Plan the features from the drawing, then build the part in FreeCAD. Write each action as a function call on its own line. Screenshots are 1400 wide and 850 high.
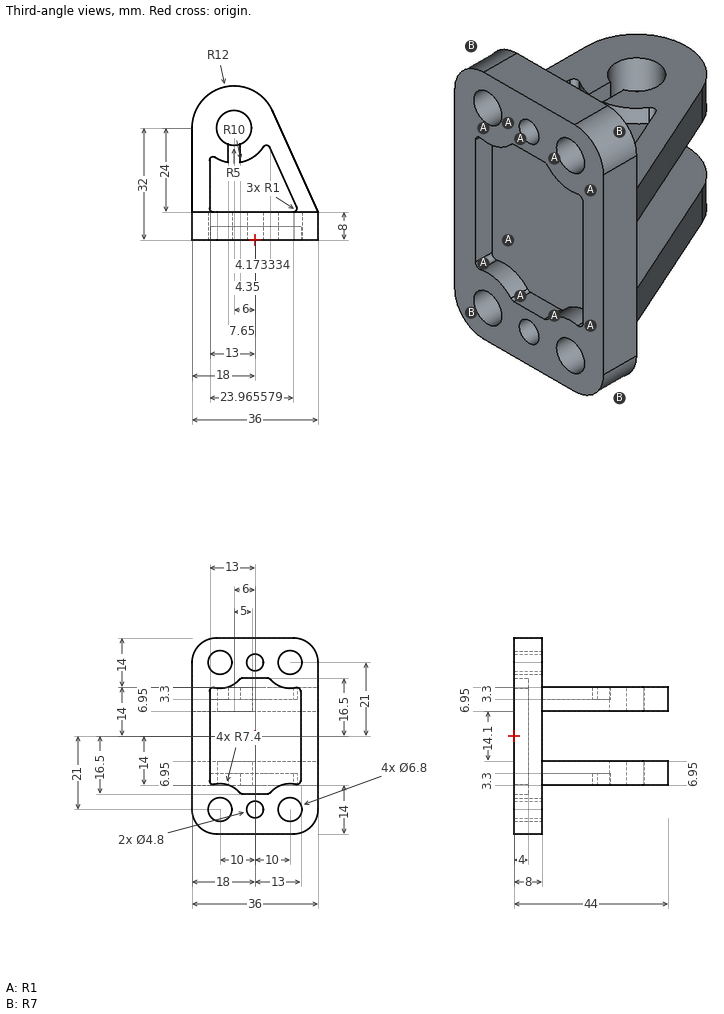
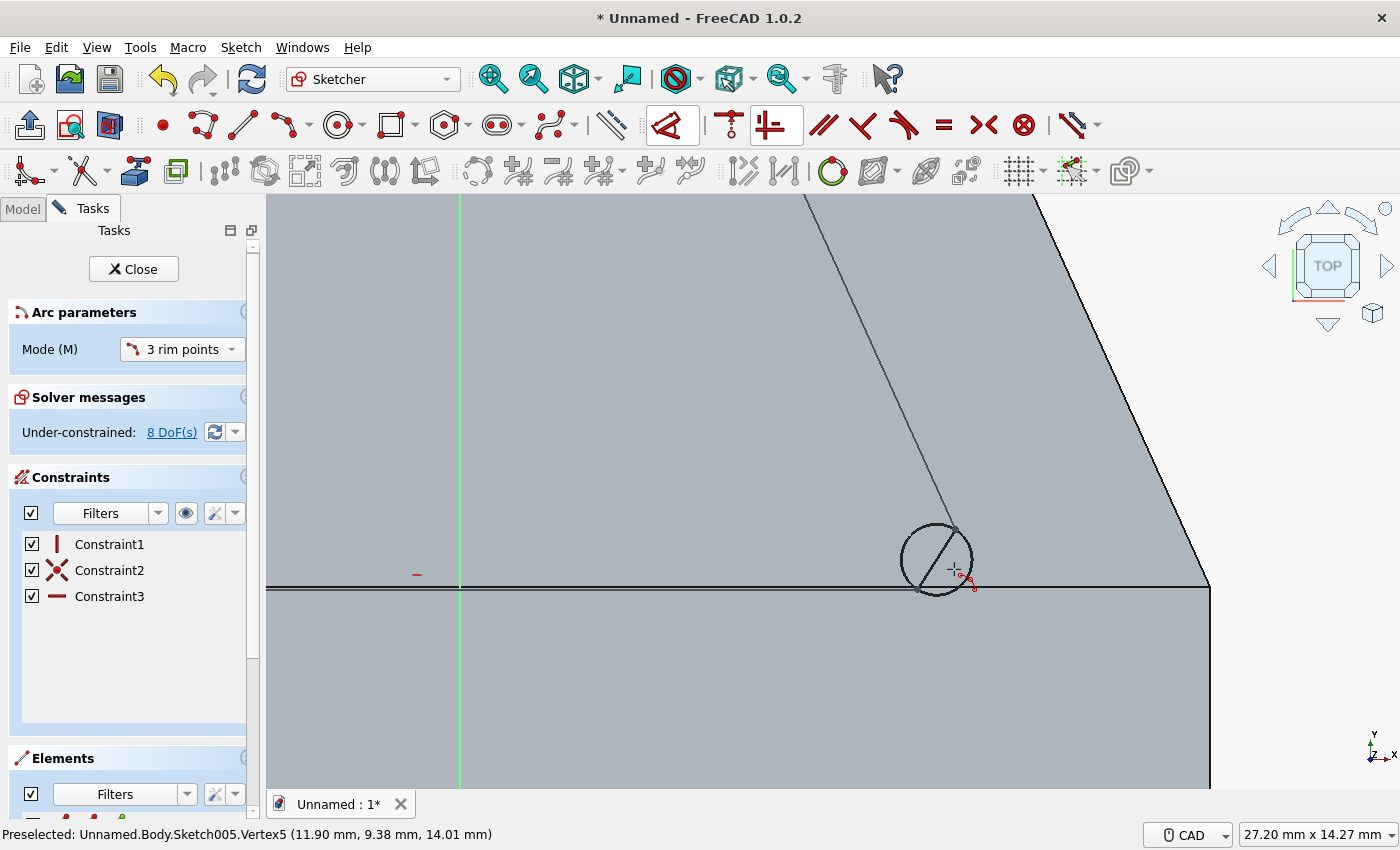
click(952, 568)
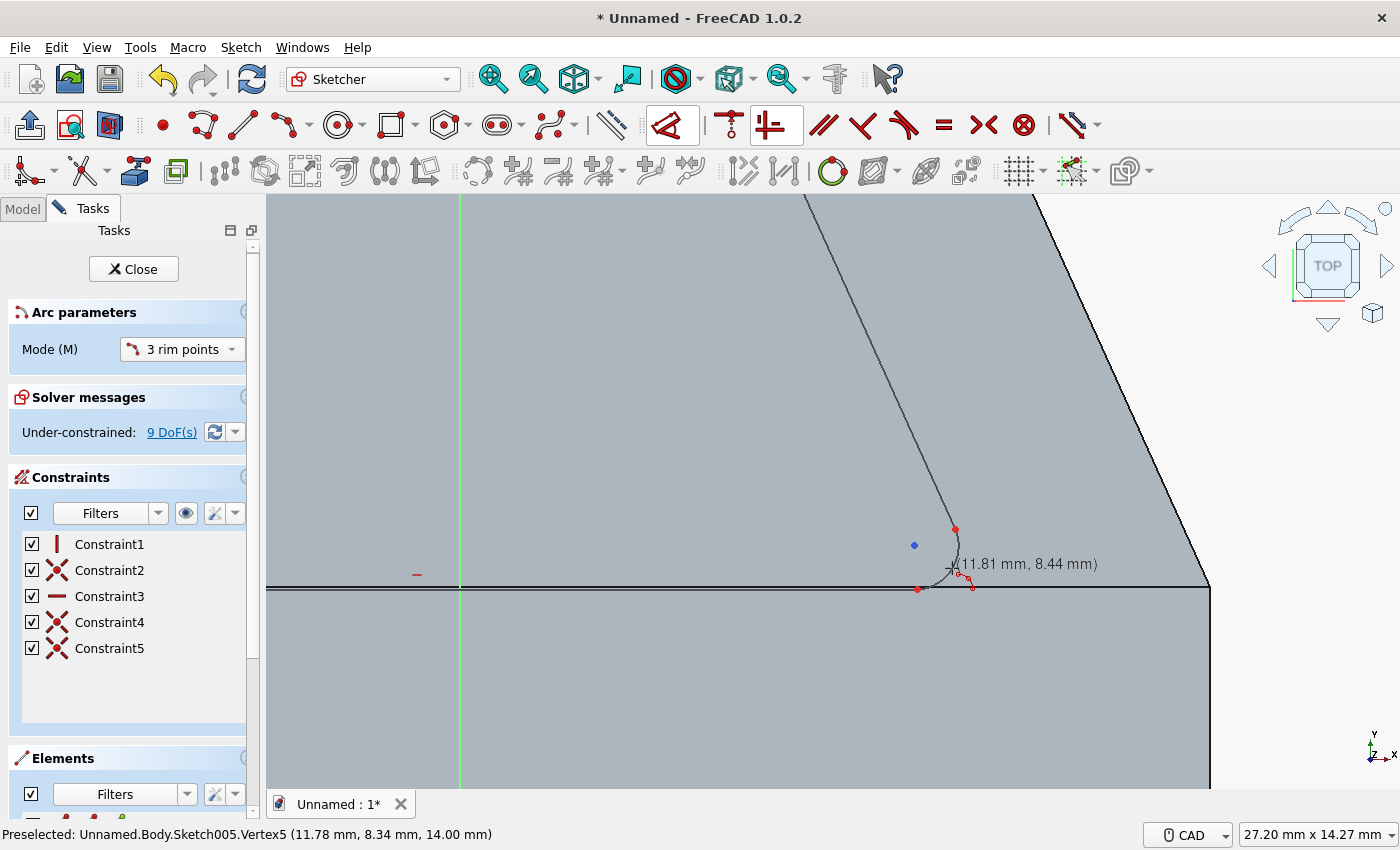
scroll(956, 570, down, 5)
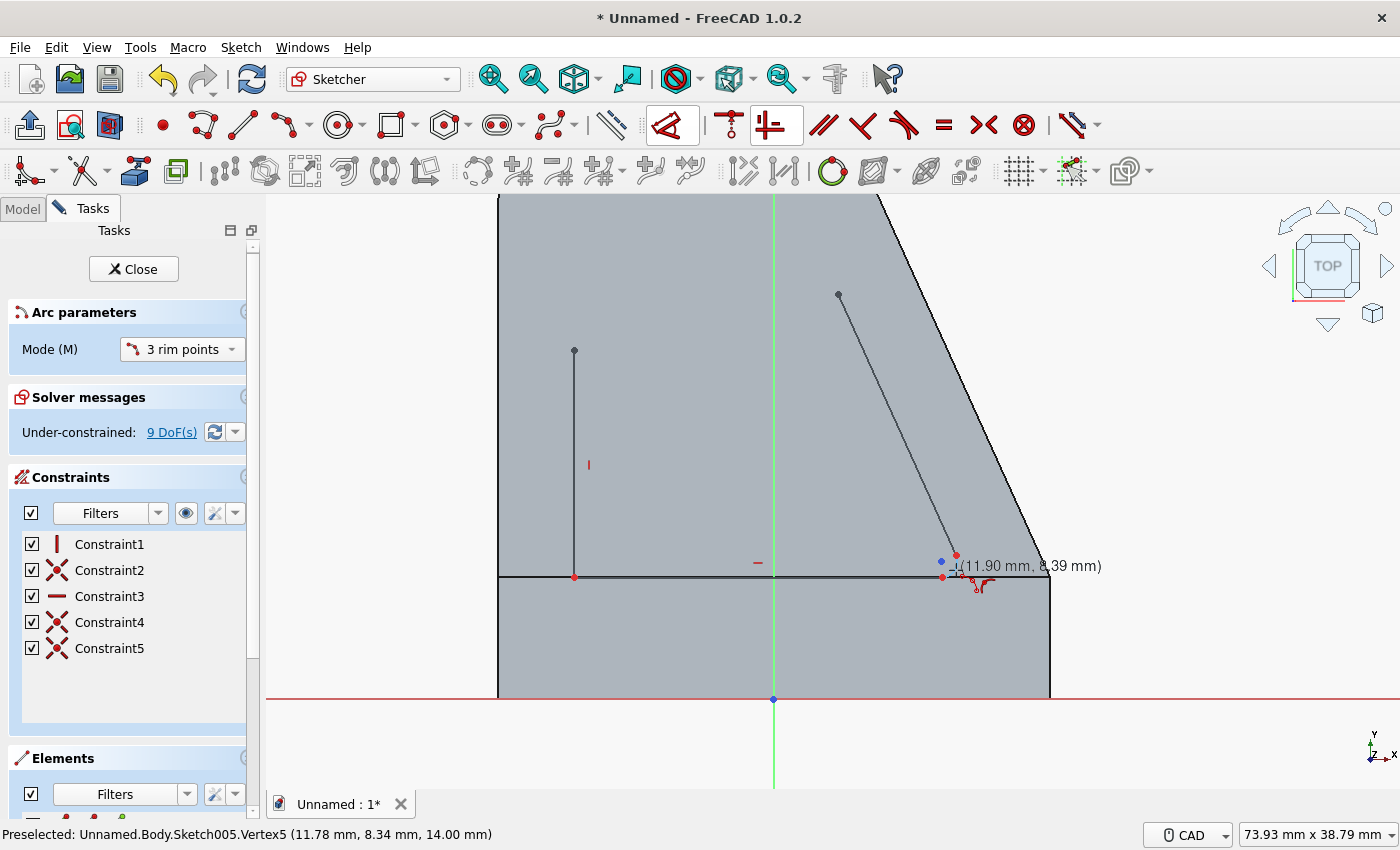
click(838, 295)
click(811, 291)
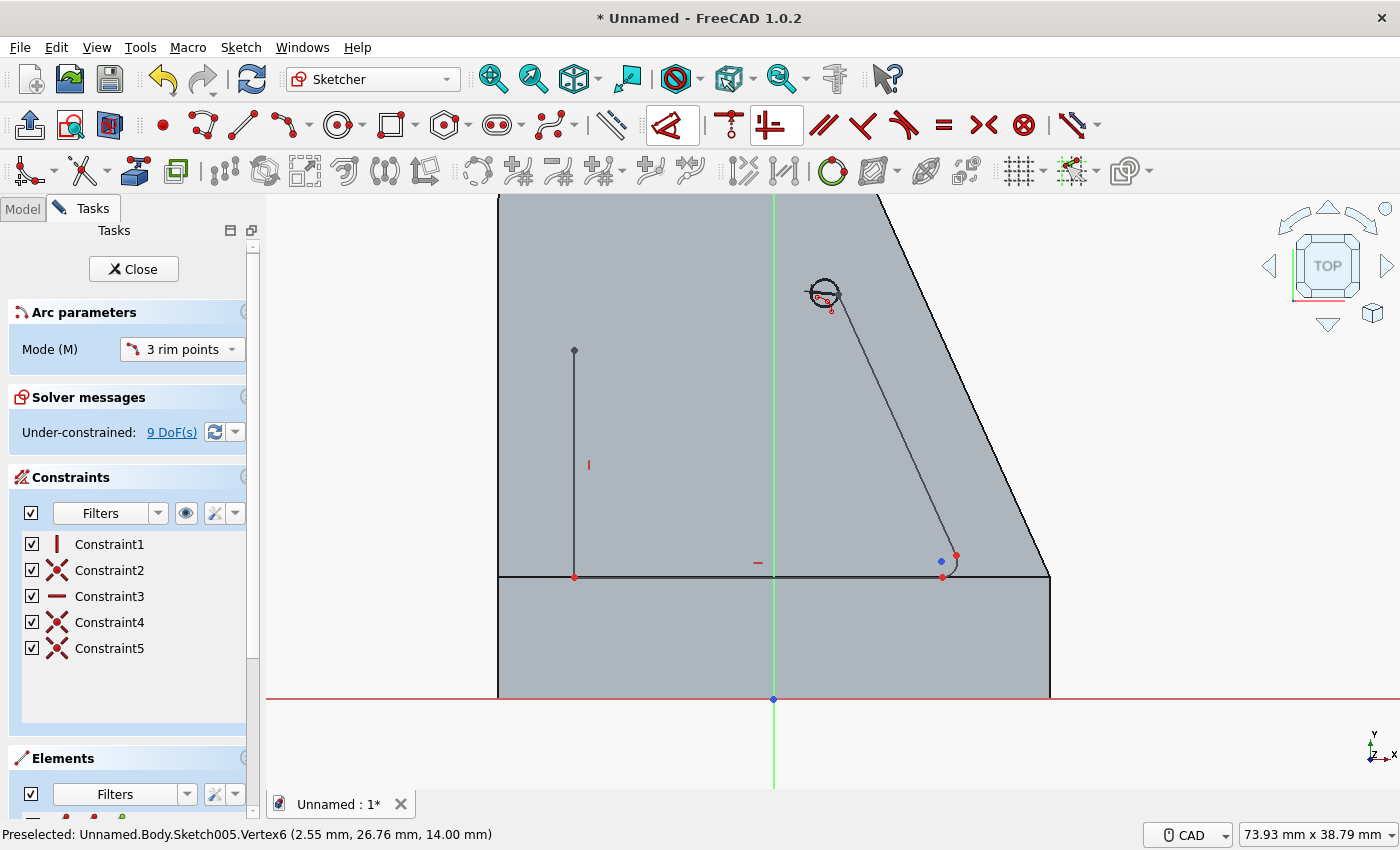
scroll(825, 284, up, 4)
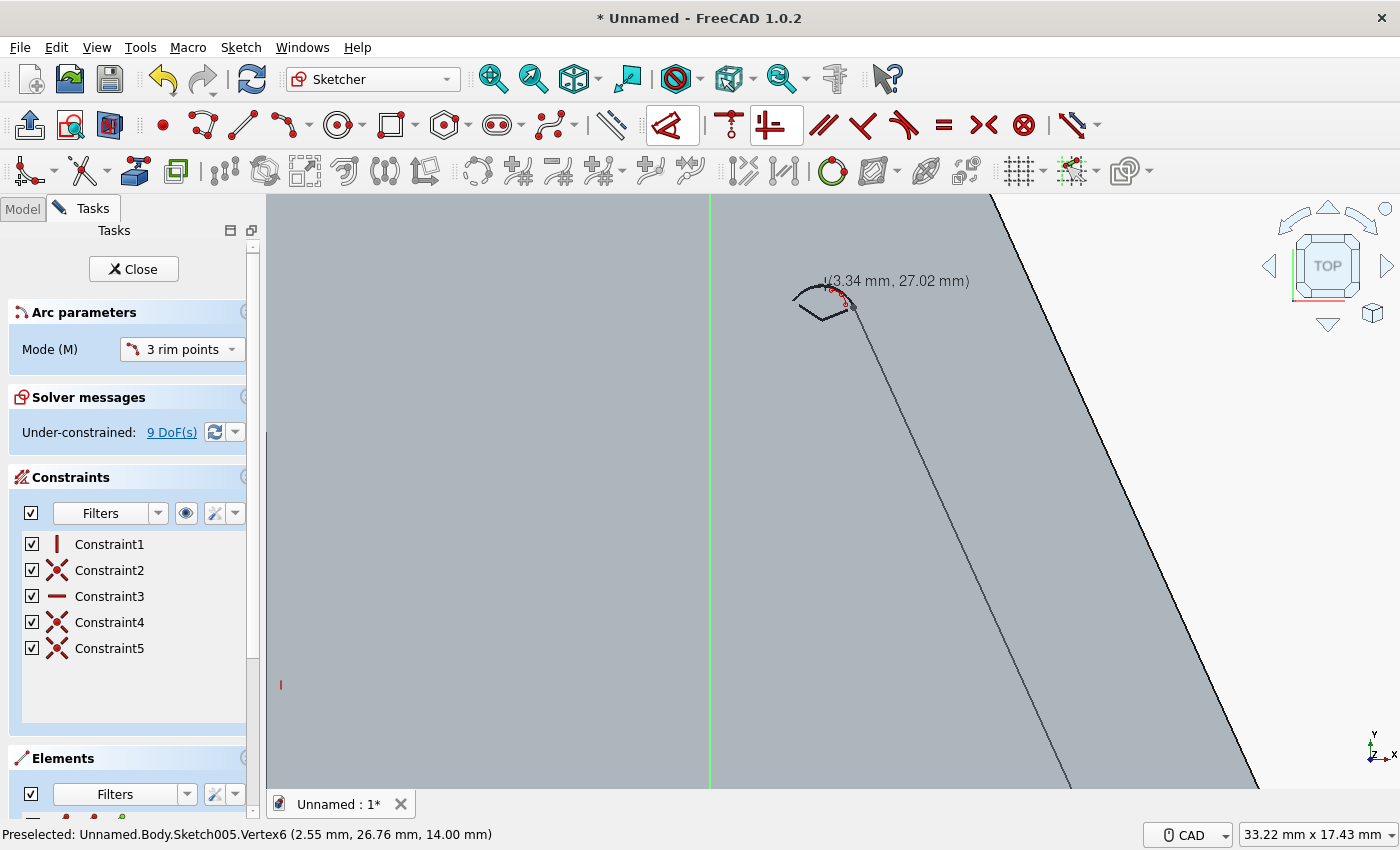
click(824, 285)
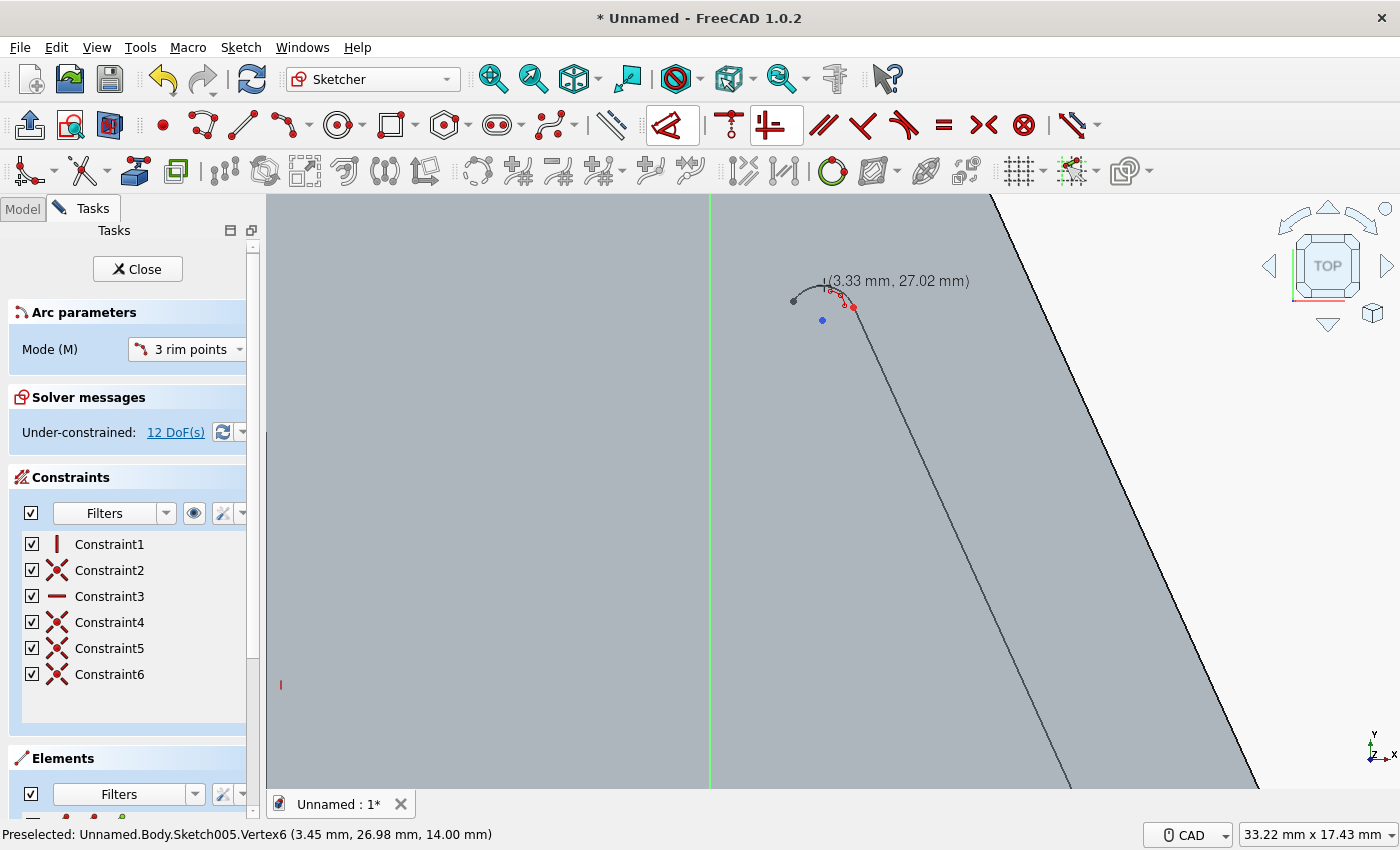
click(793, 302)
click(319, 402)
click(577, 450)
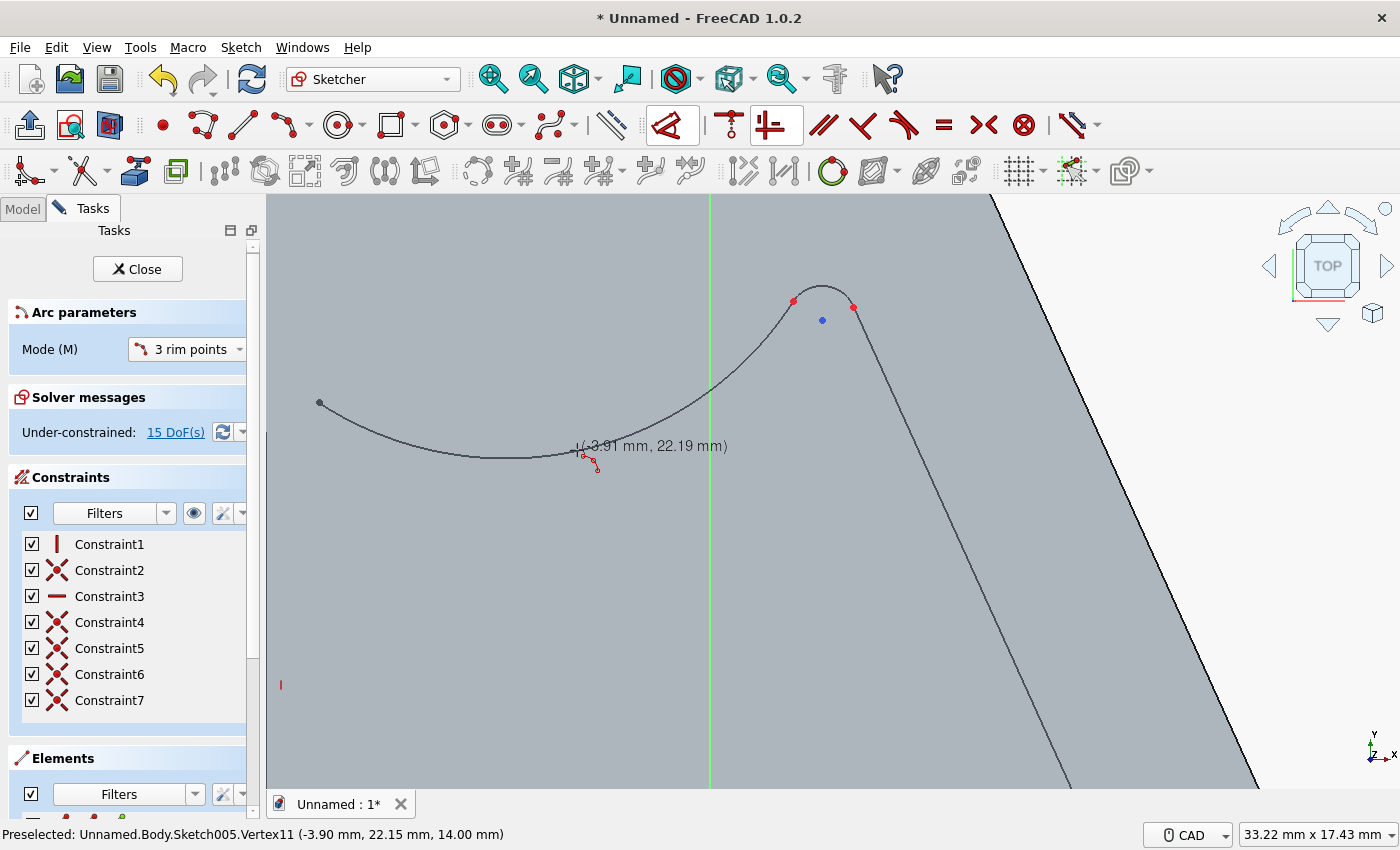
click(319, 403)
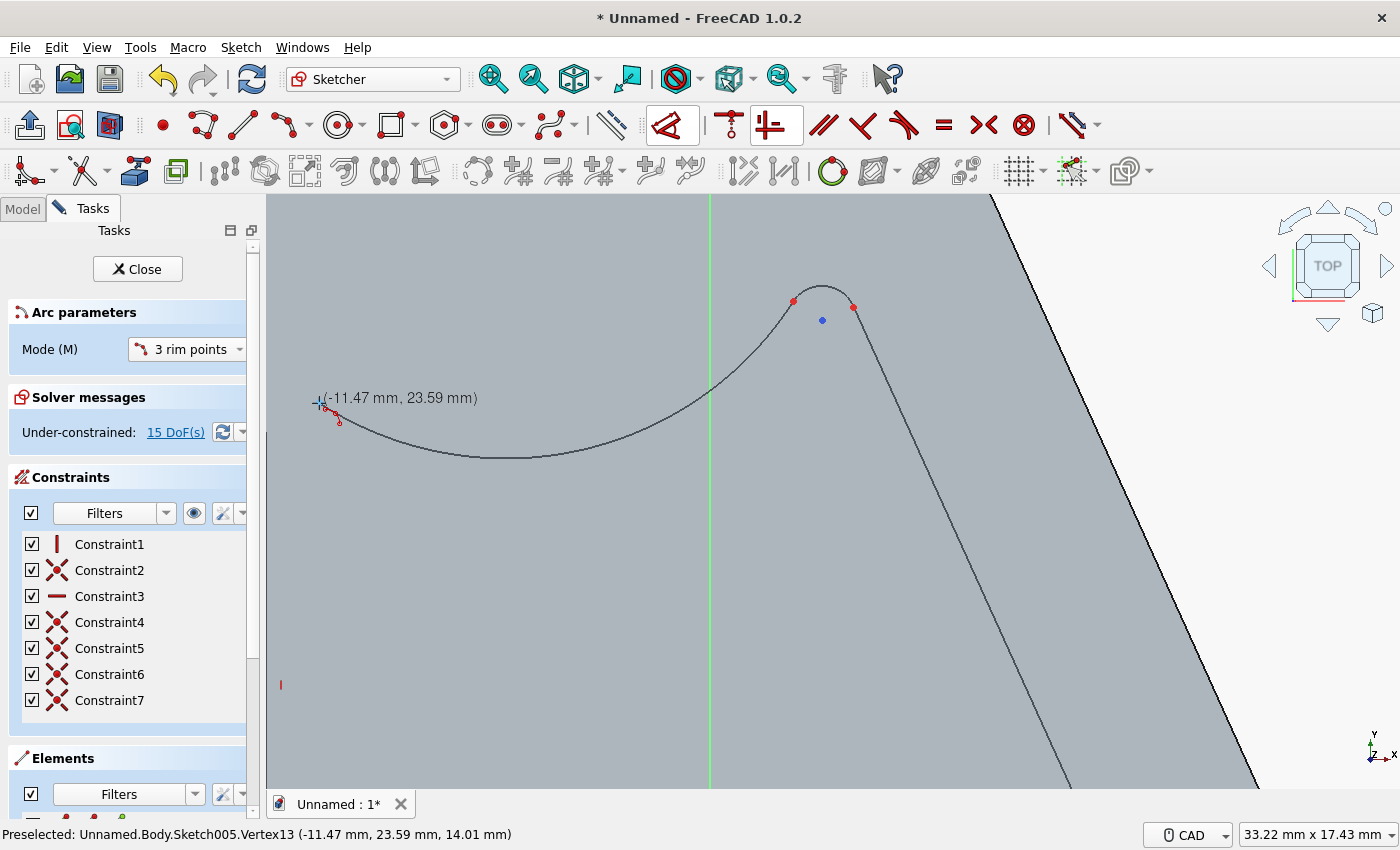
scroll(824, 283, down, 4)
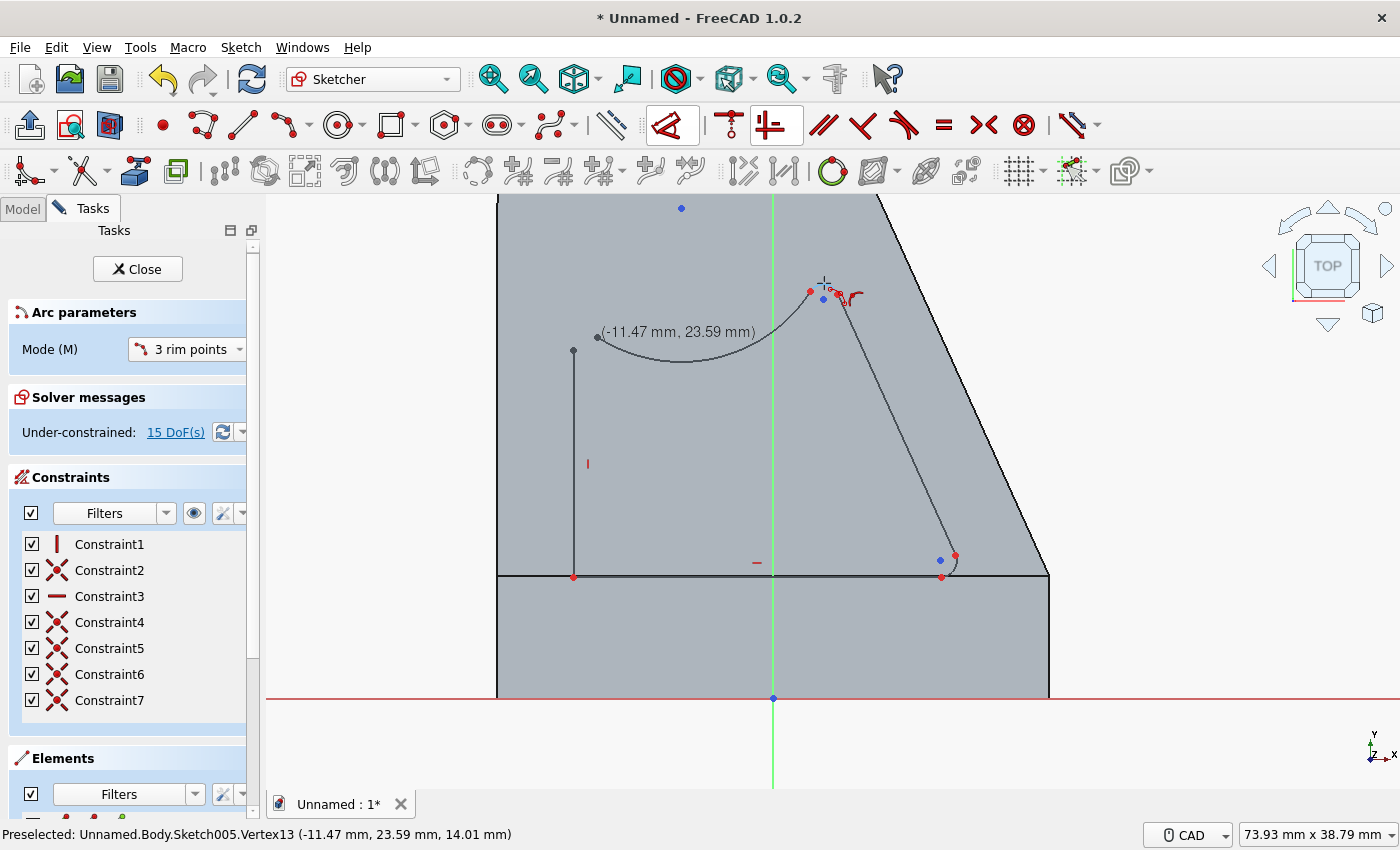
click(574, 350)